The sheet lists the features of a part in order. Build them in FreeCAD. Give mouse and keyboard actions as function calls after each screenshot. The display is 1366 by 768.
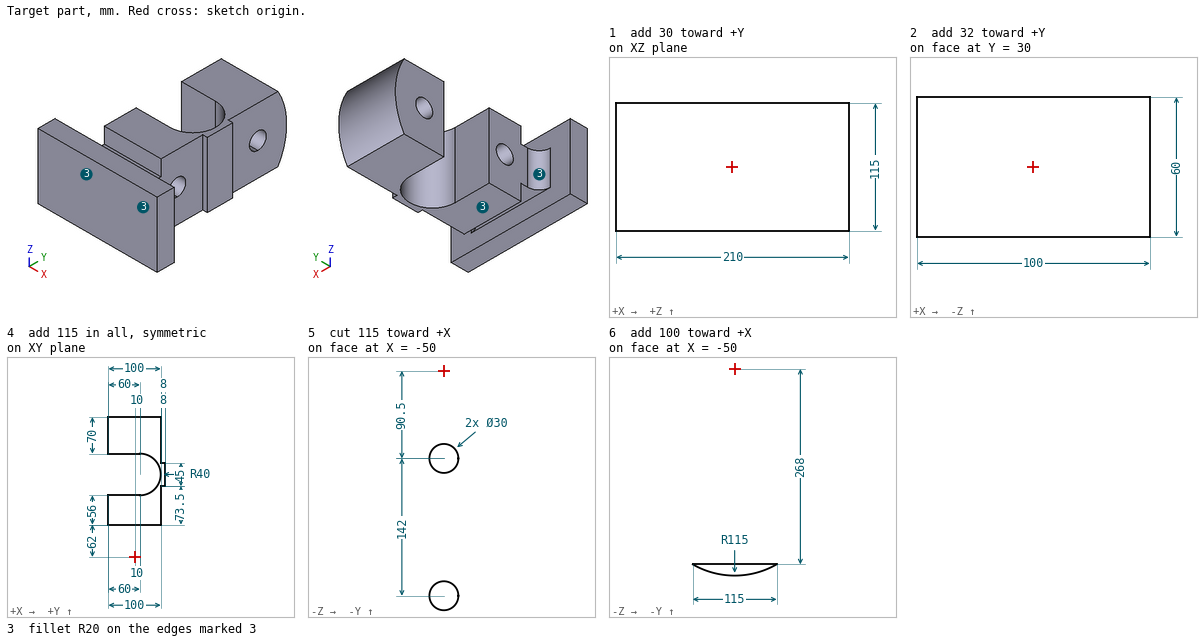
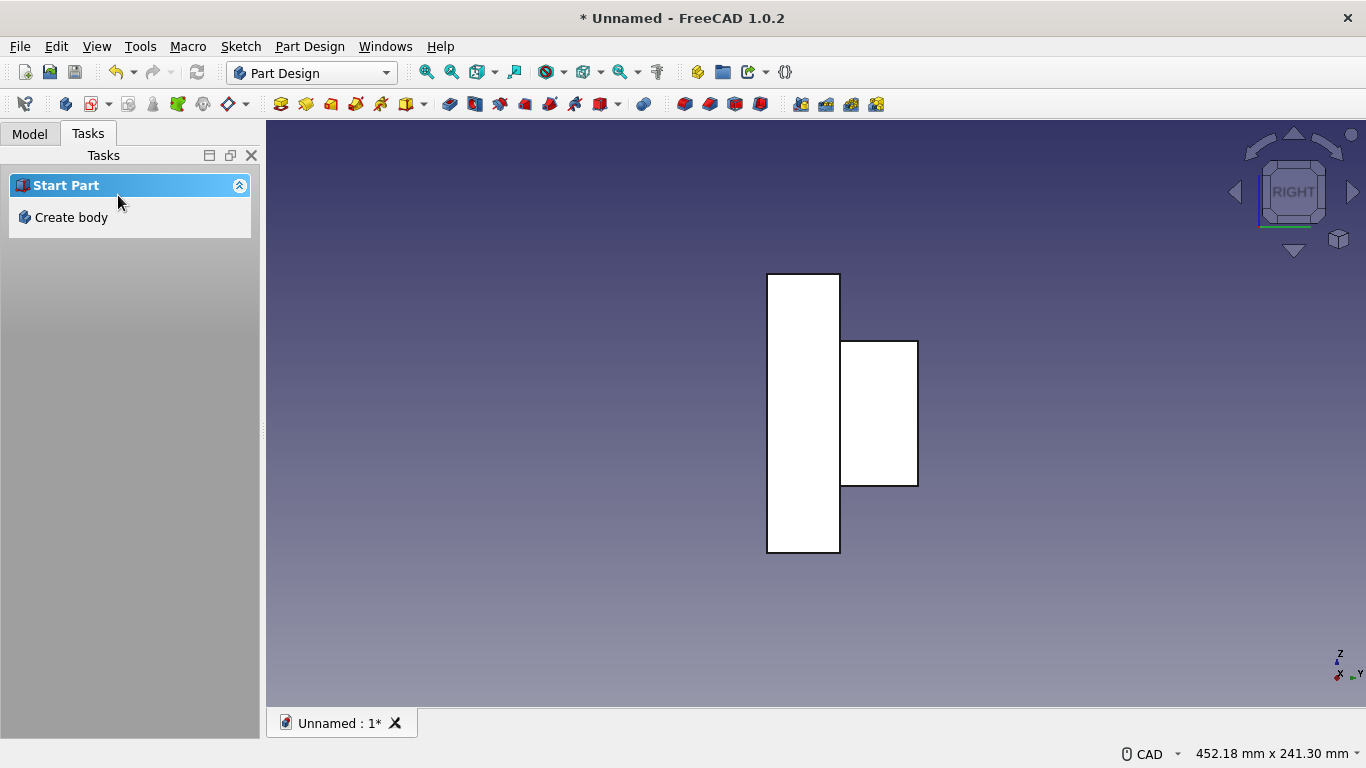
key(5)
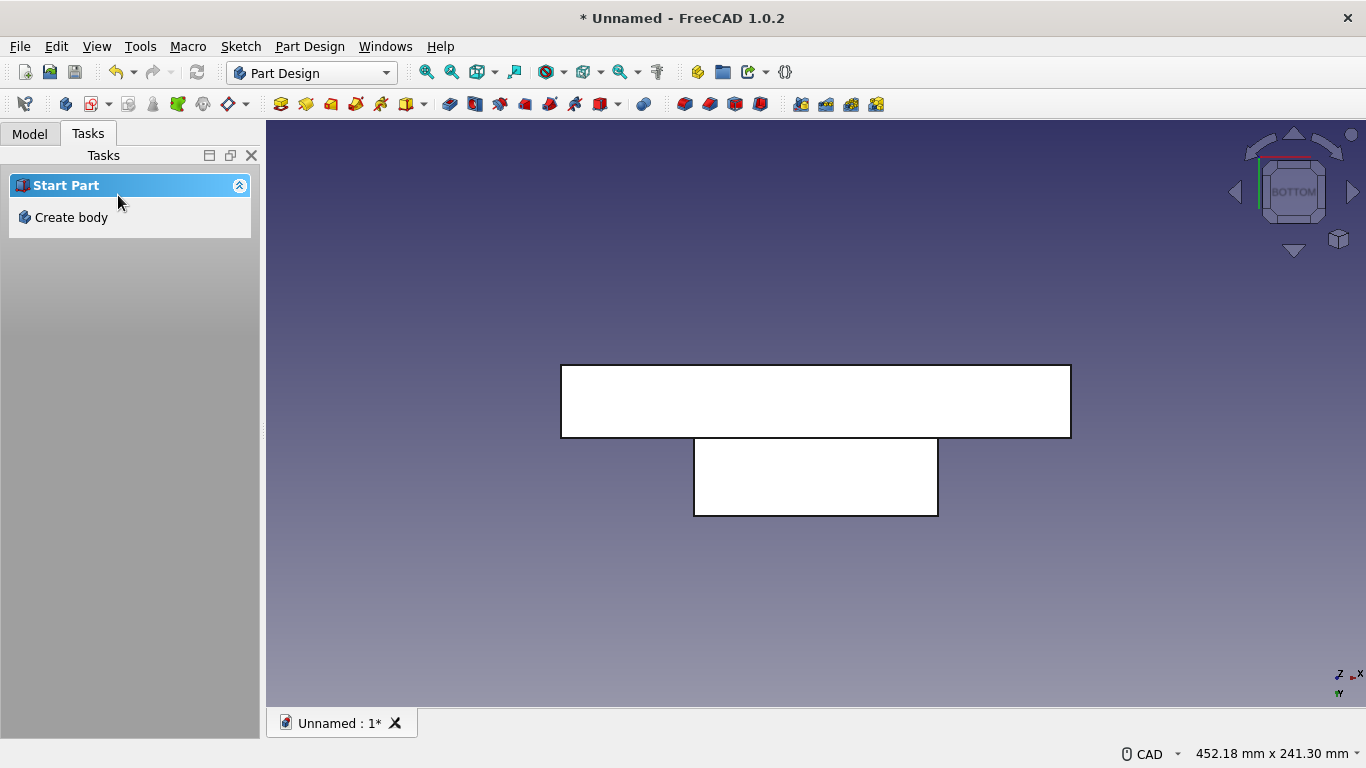
key(4)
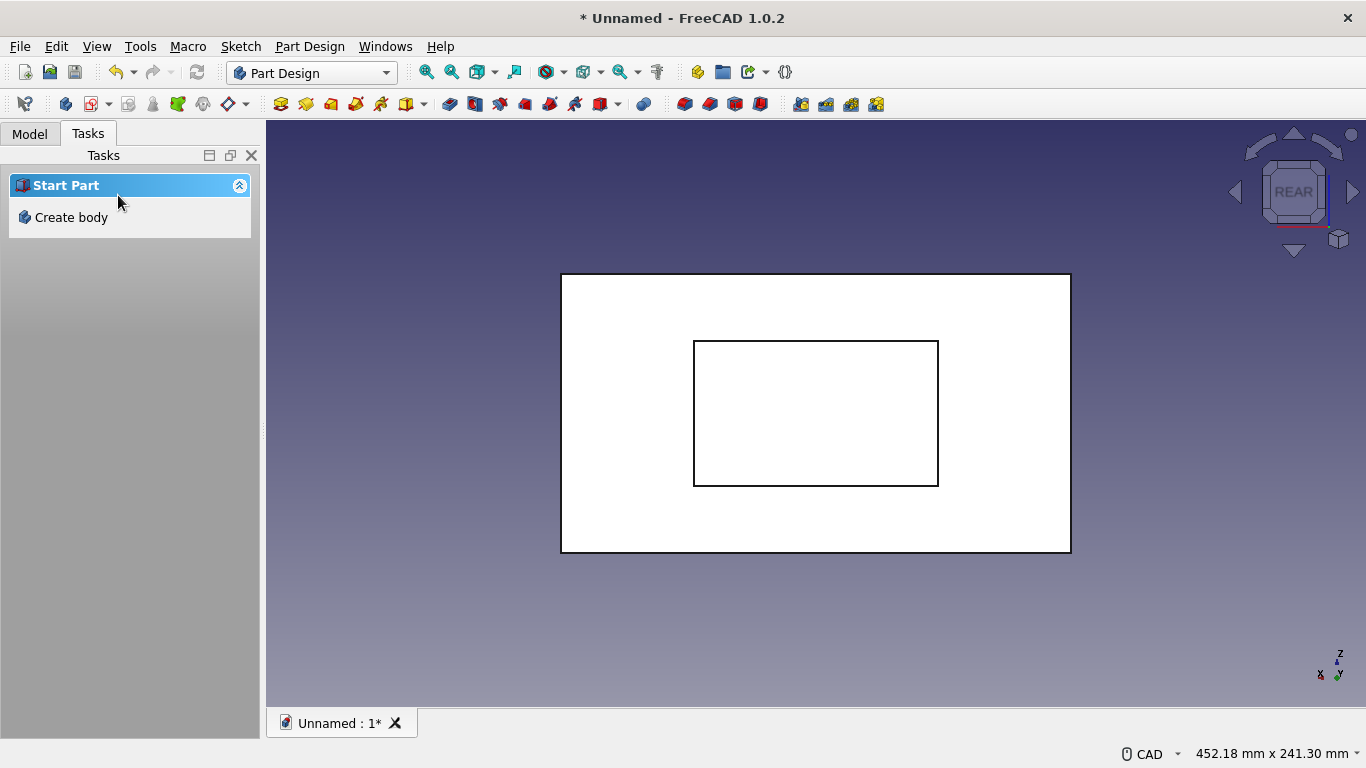
key(6)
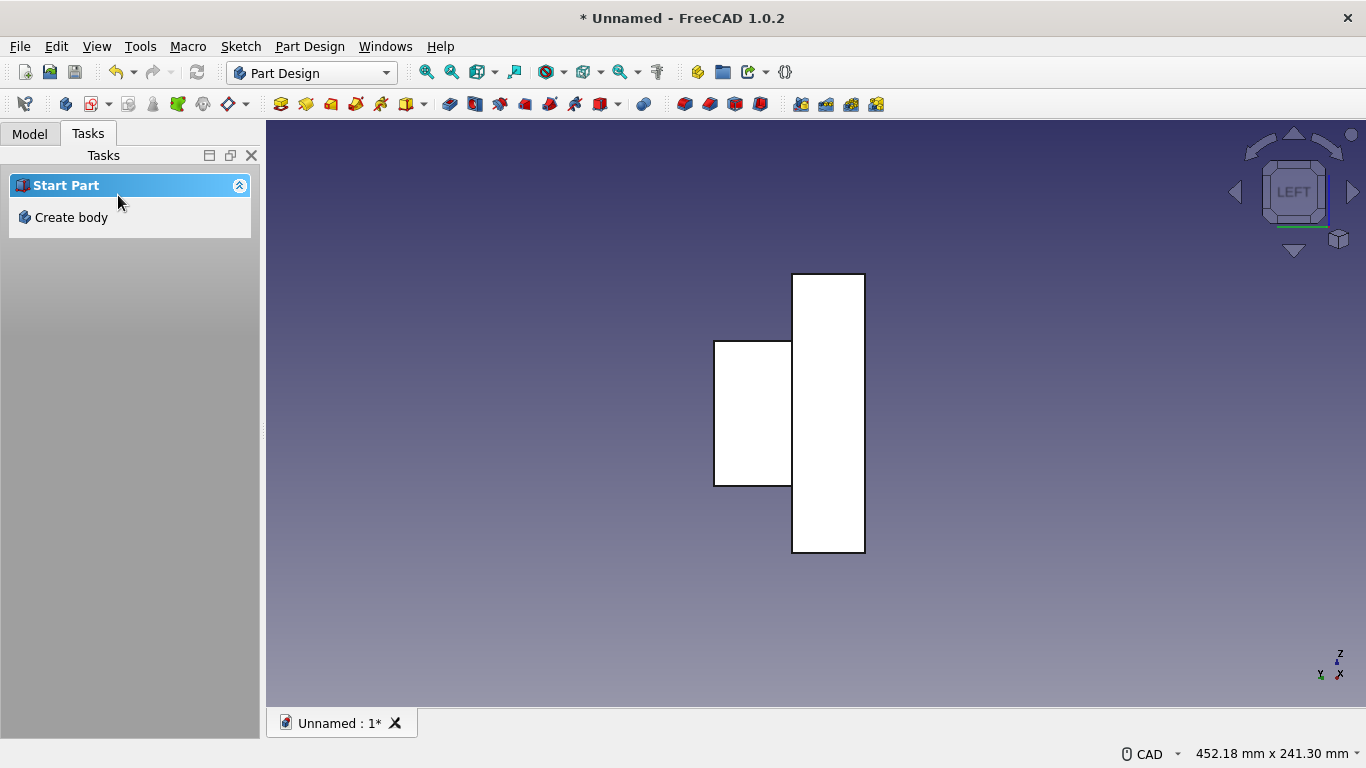
key(v)
key(3)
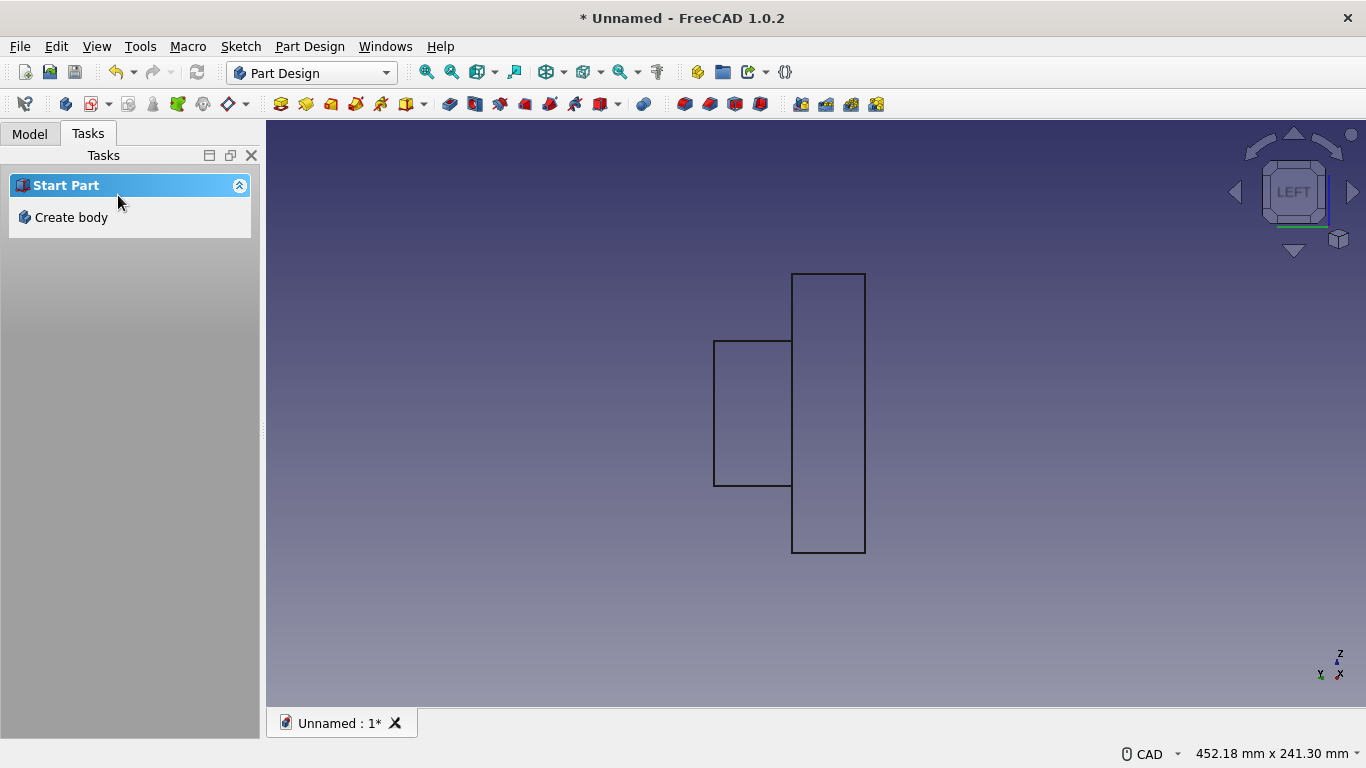
key(0)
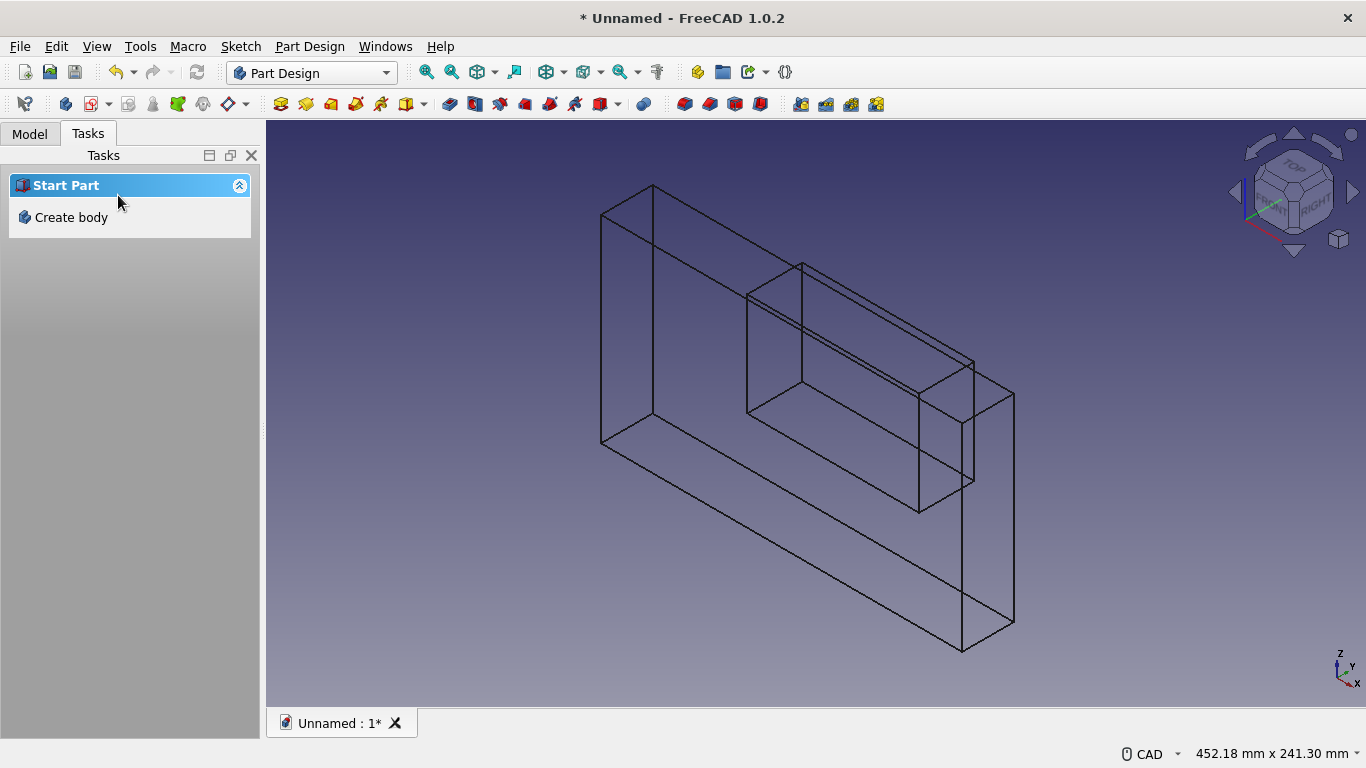
click(919, 452)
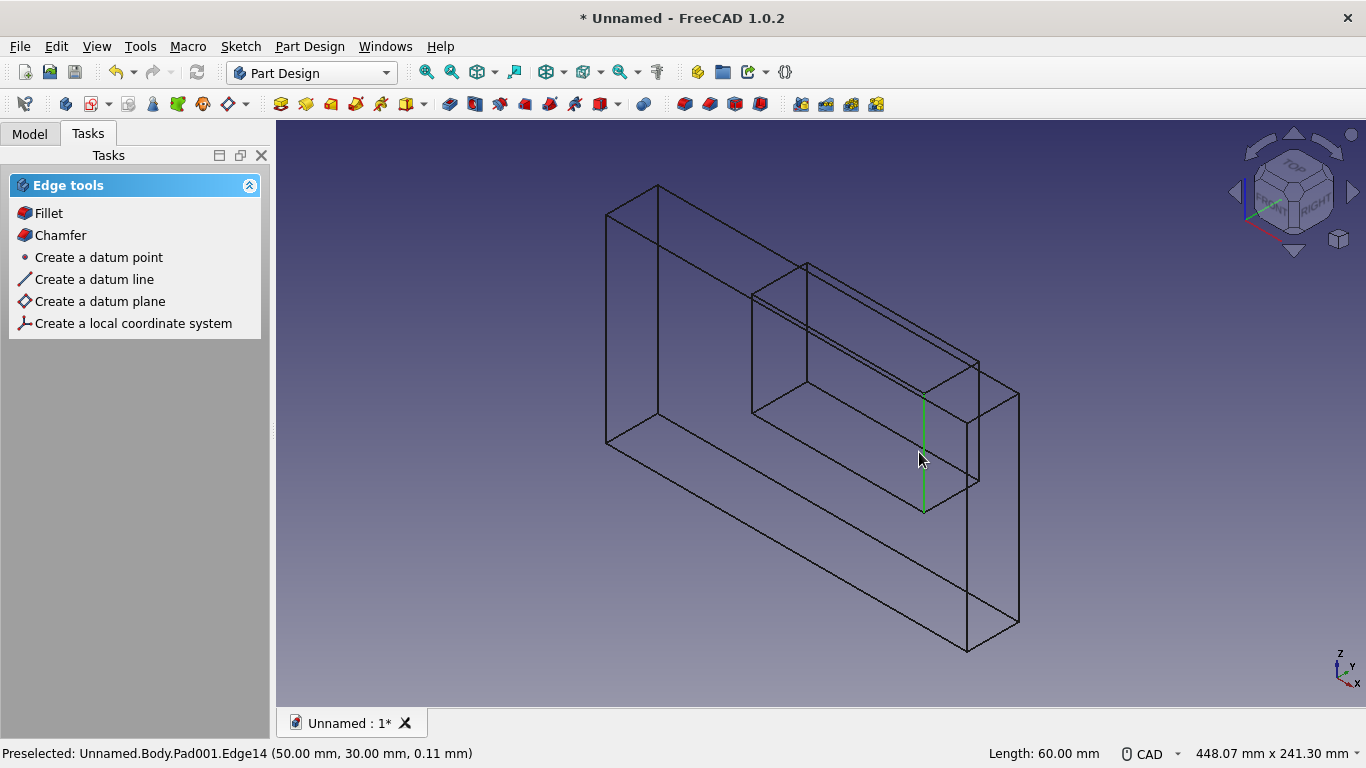
click(752, 353, ctrl)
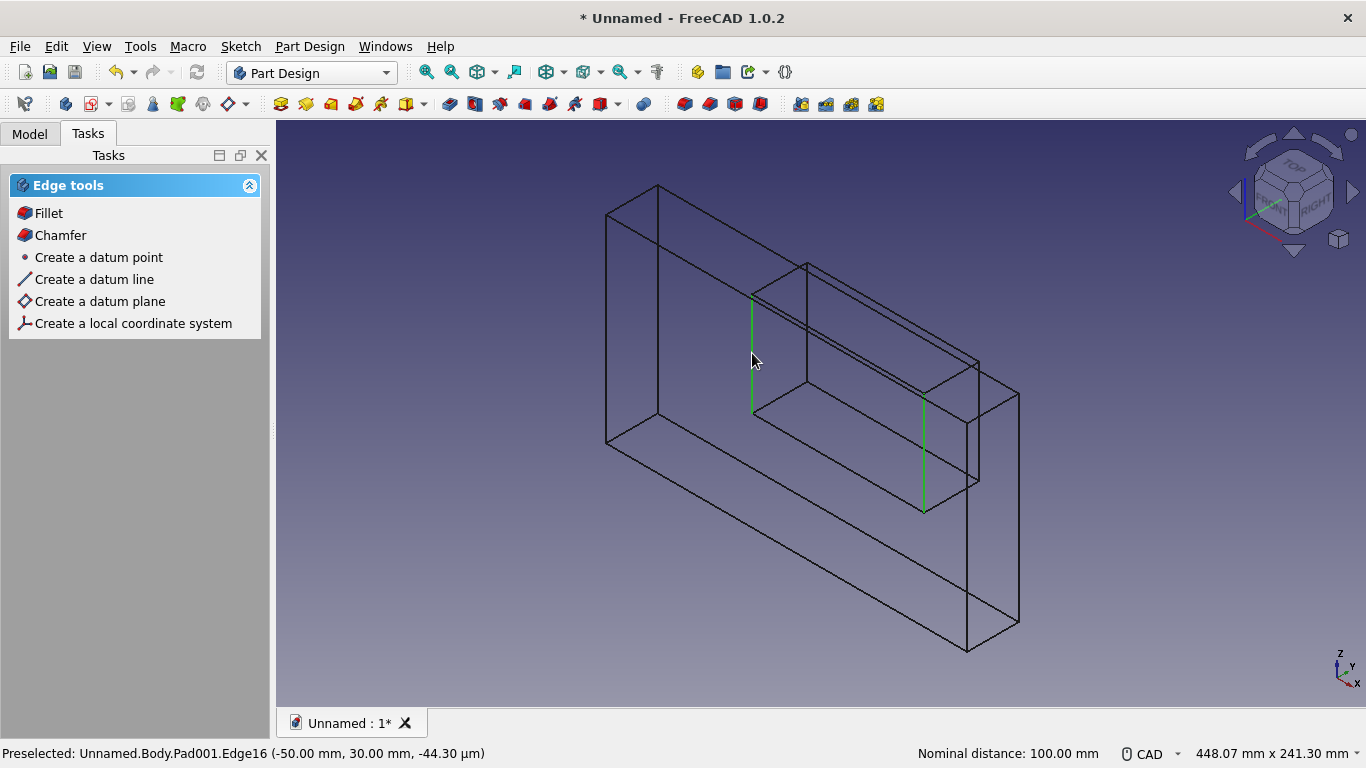
key(v)
key(1)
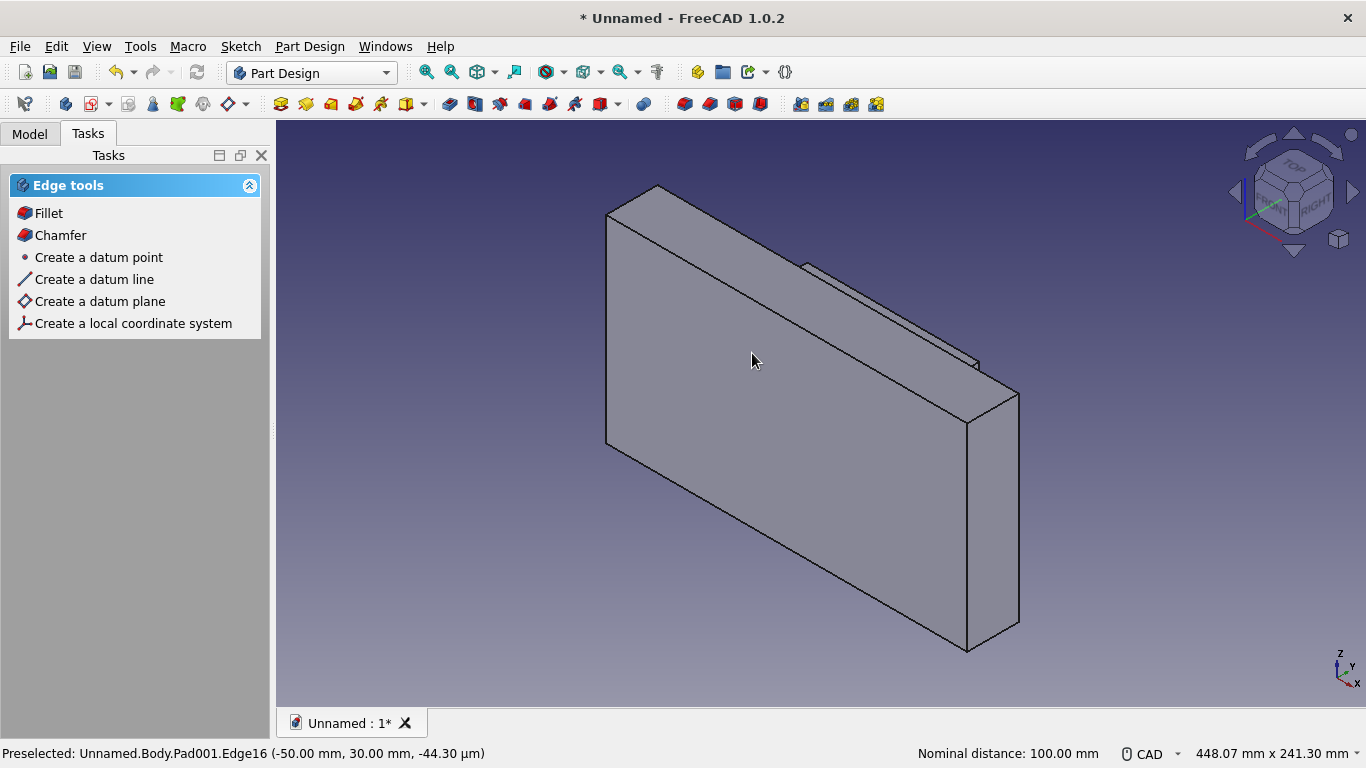
click(685, 104)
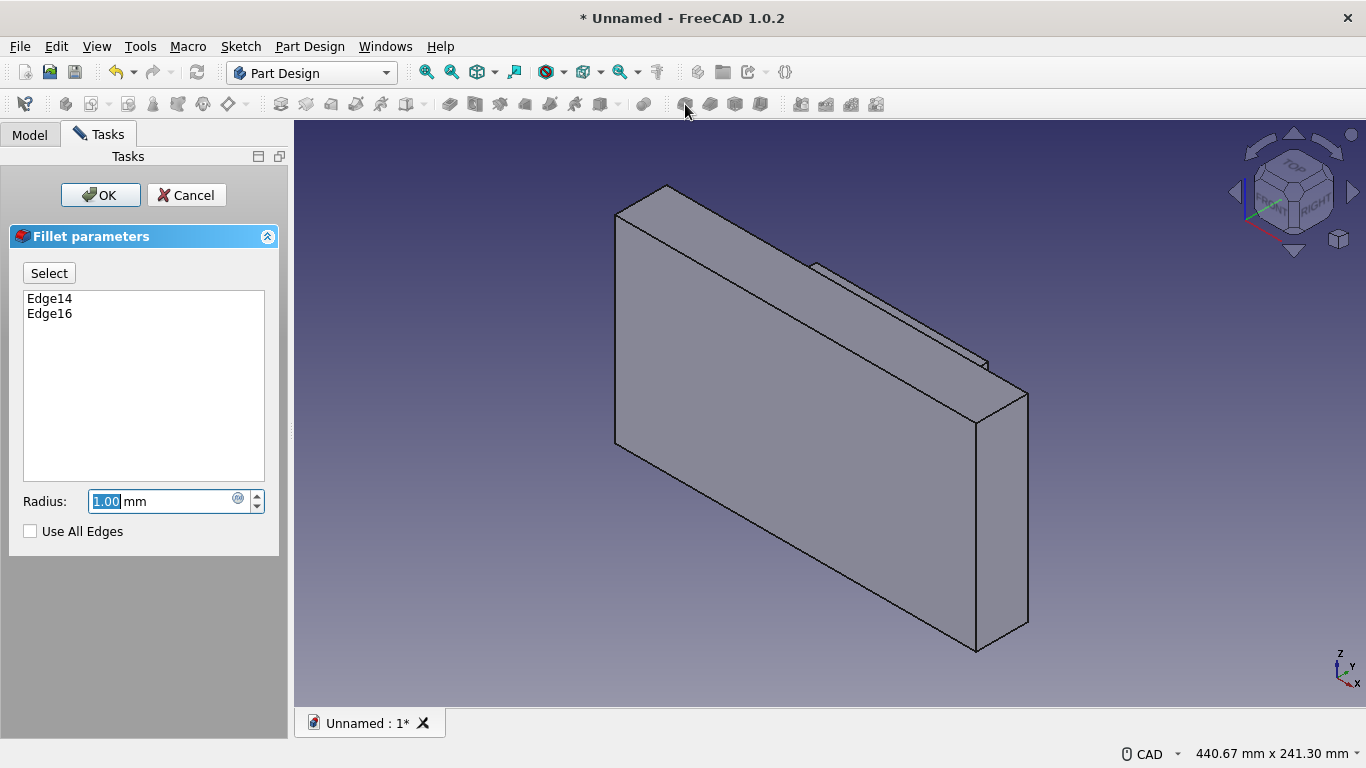
text(20)
key(Tab)